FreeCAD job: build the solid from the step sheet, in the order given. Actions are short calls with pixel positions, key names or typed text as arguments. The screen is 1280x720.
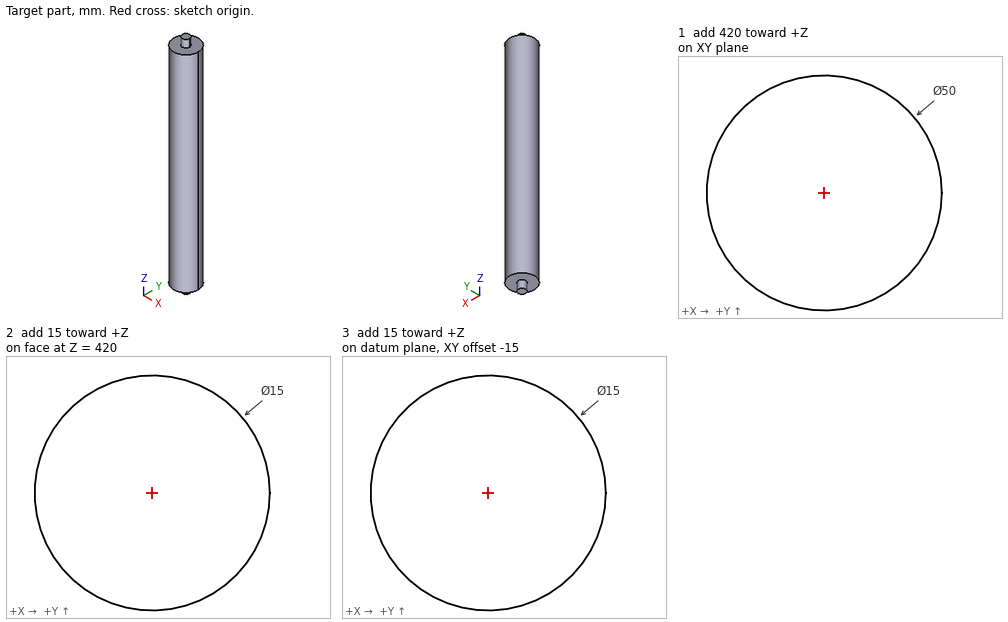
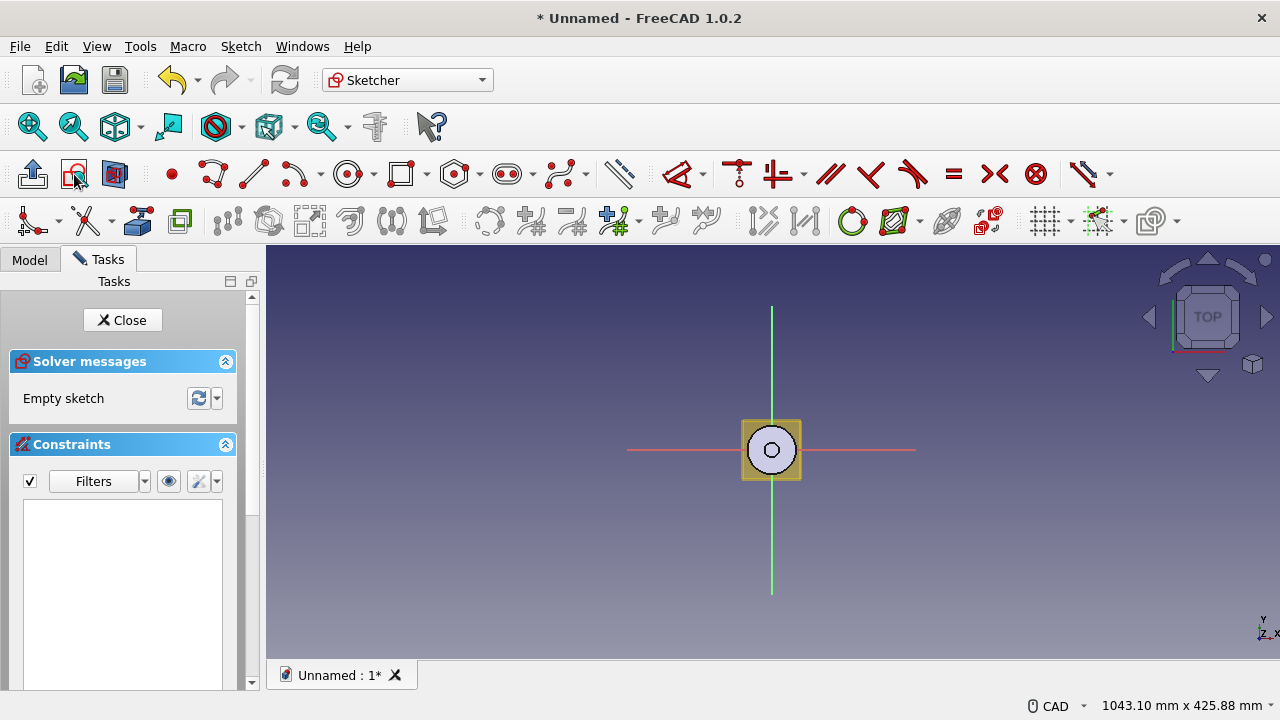
key(q)
key(s)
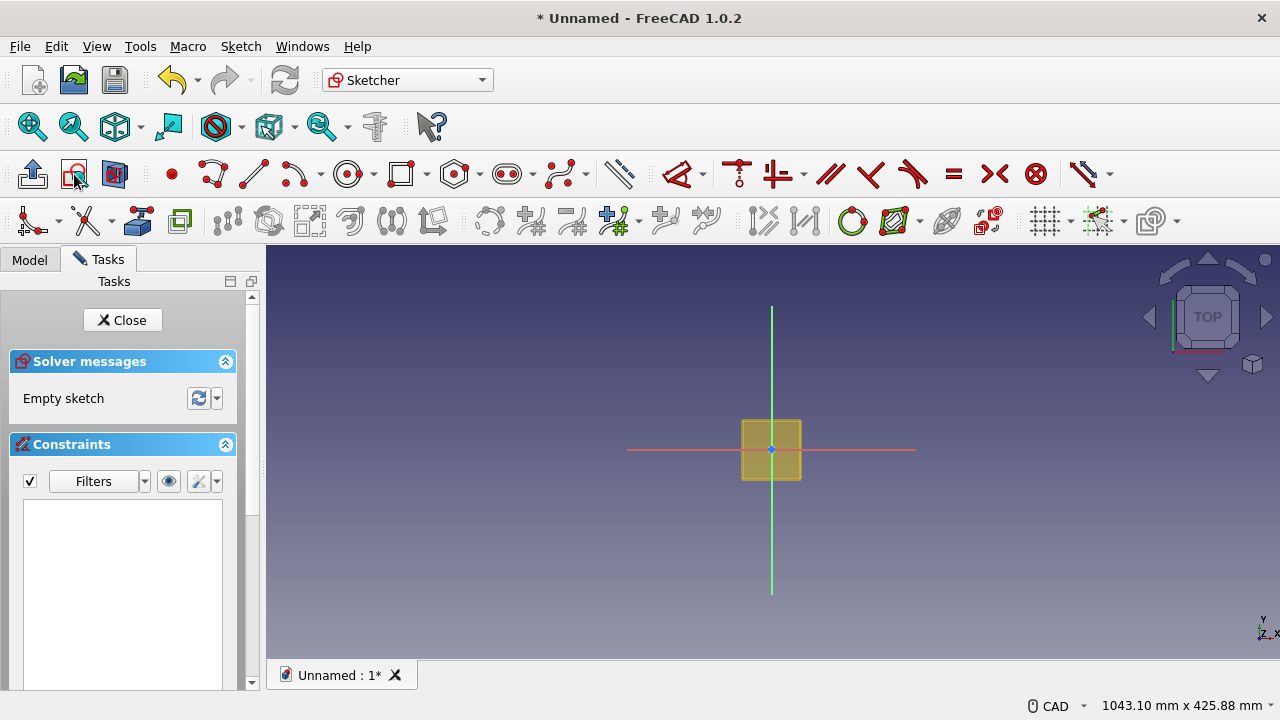
scroll(776, 450, up, 14)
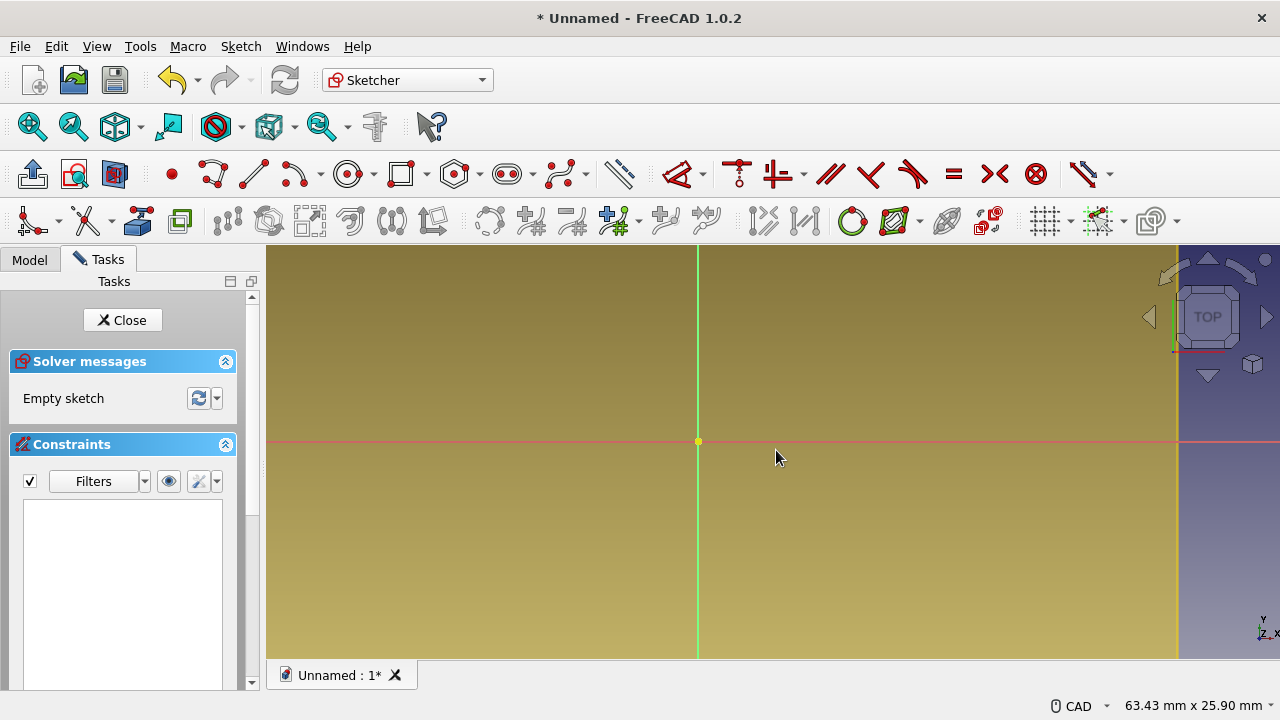
key(g)
key(c)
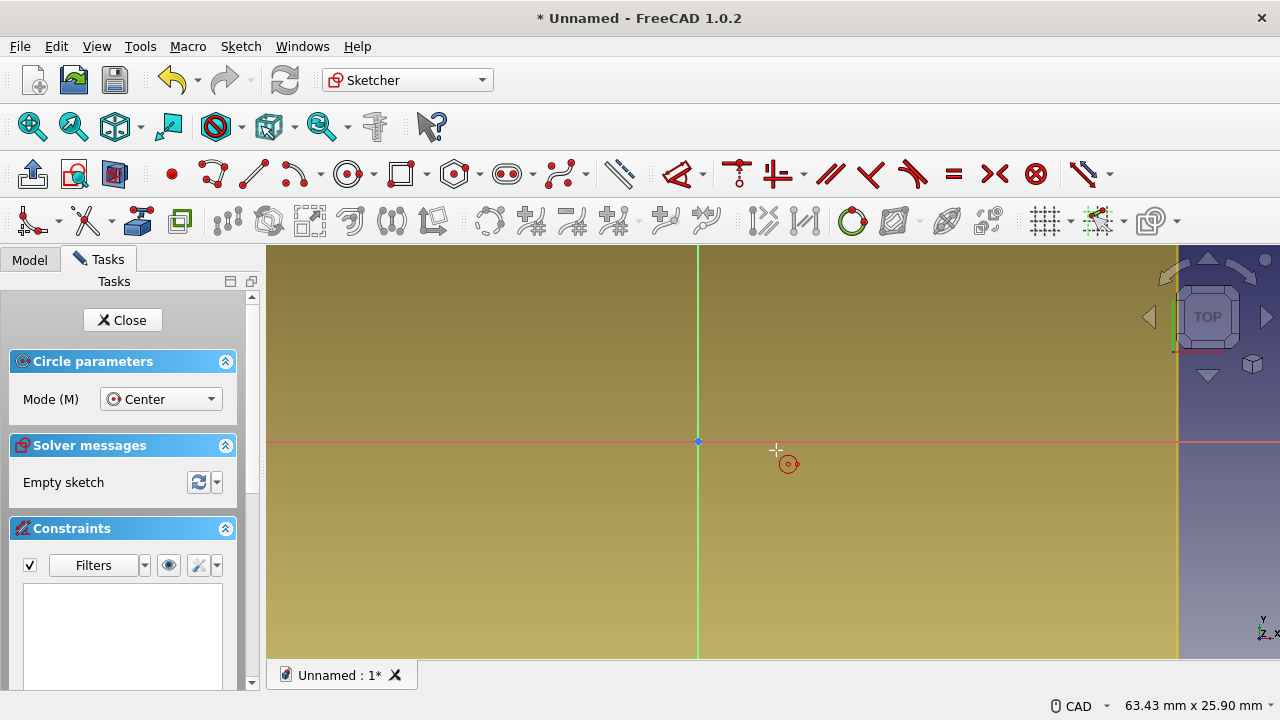
click(698, 442)
move(783, 357)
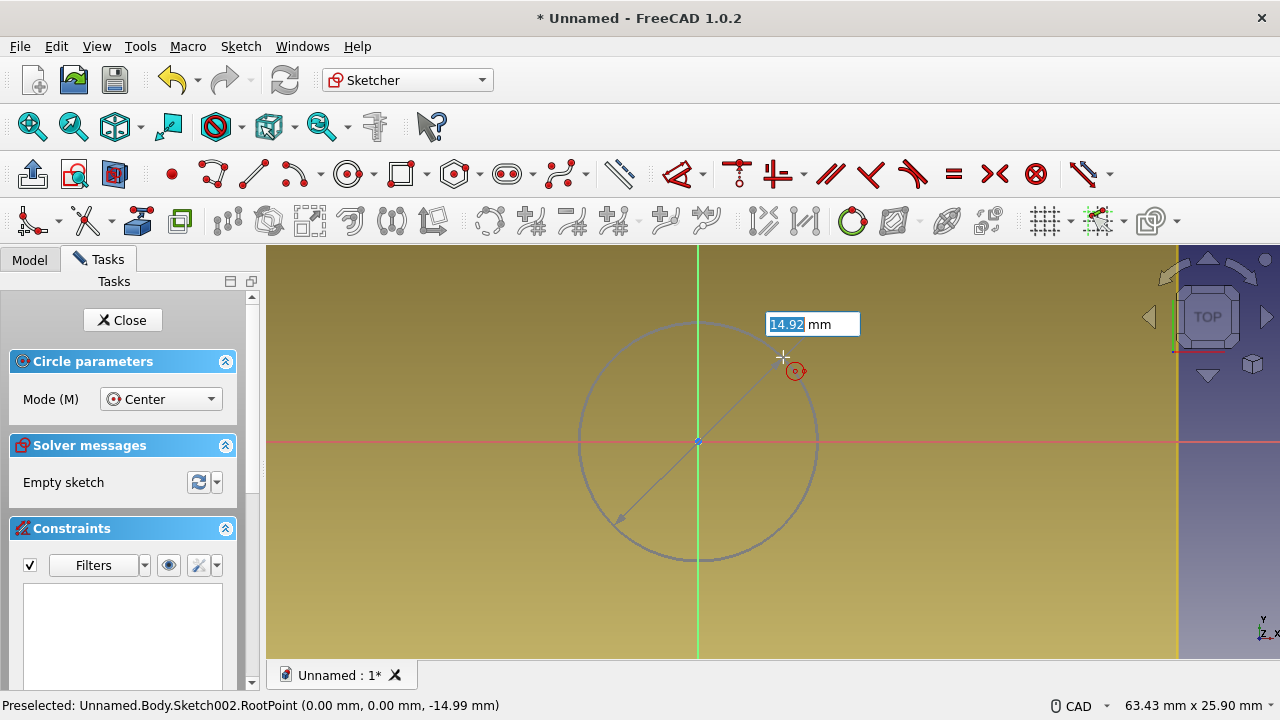
text(15)
key(Return)
key(Escape)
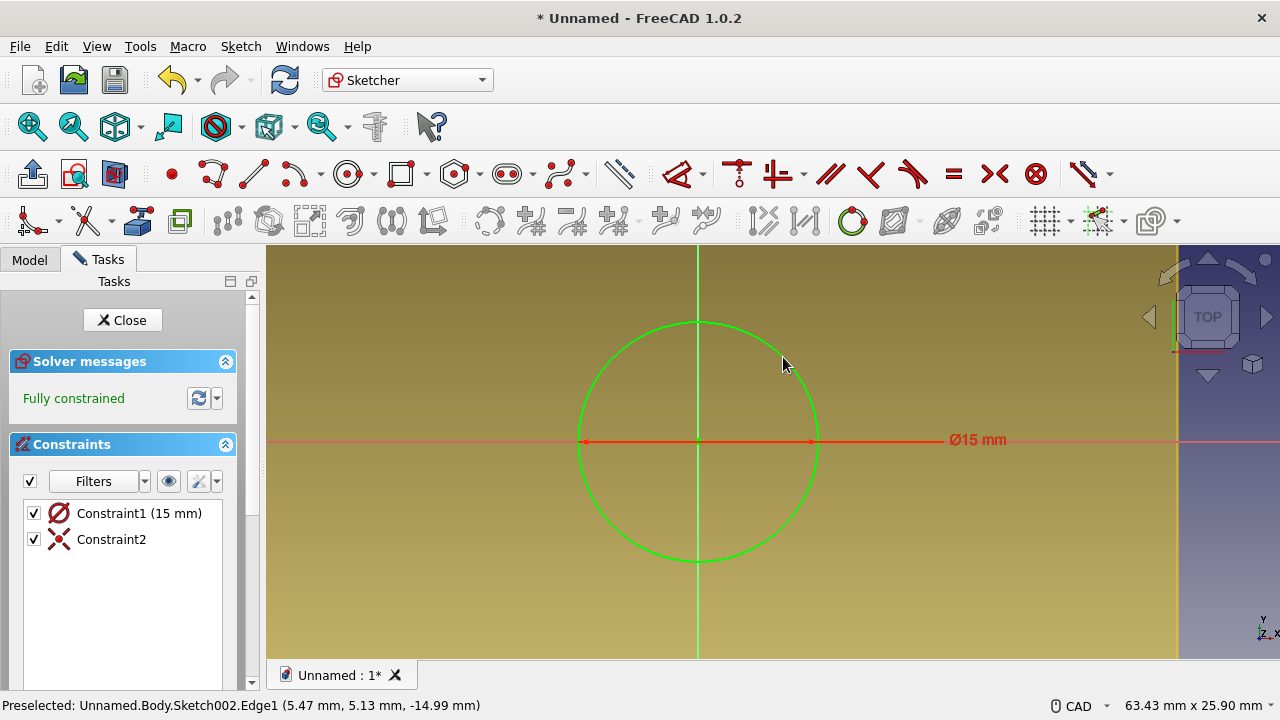
click(123, 320)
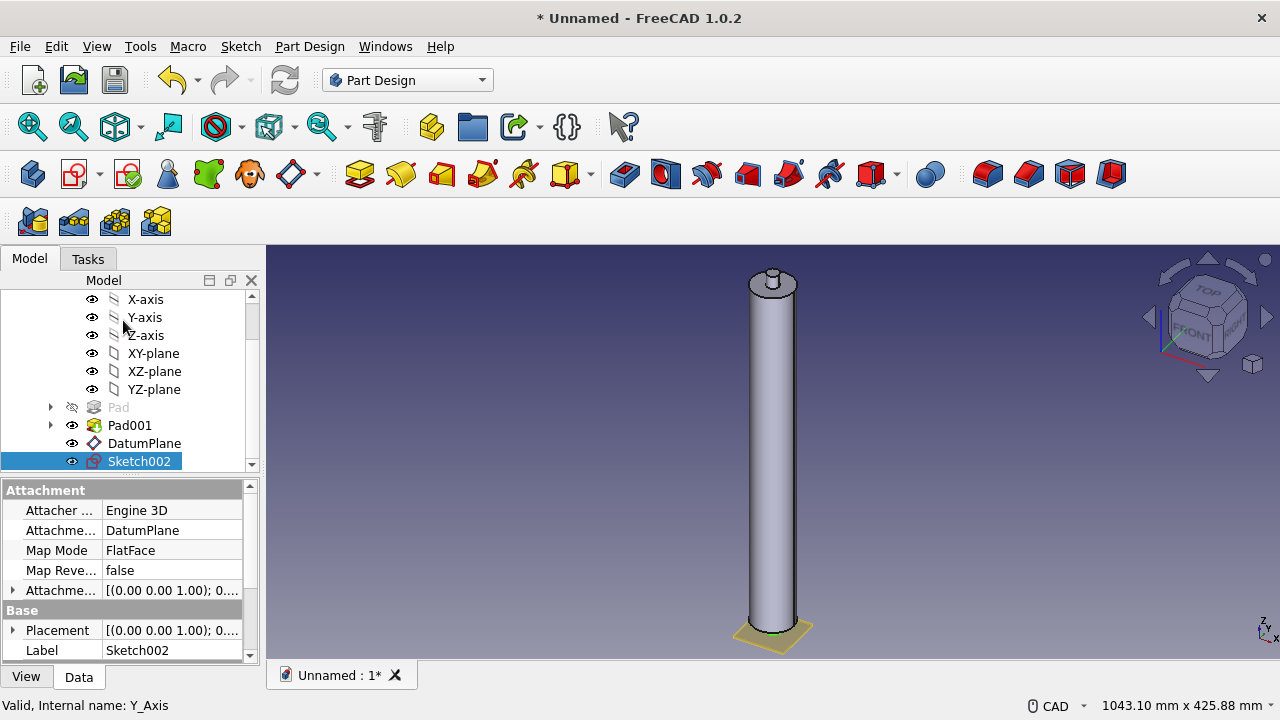
click(360, 174)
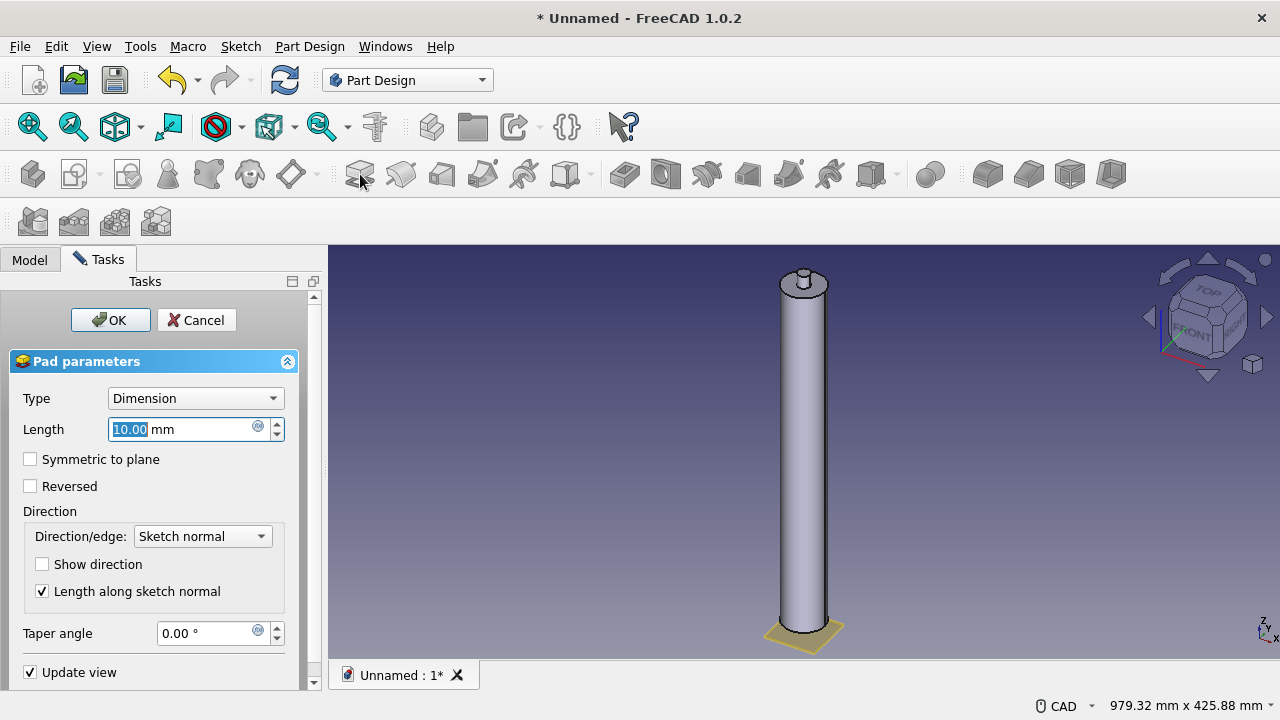
text(15)
key(Tab)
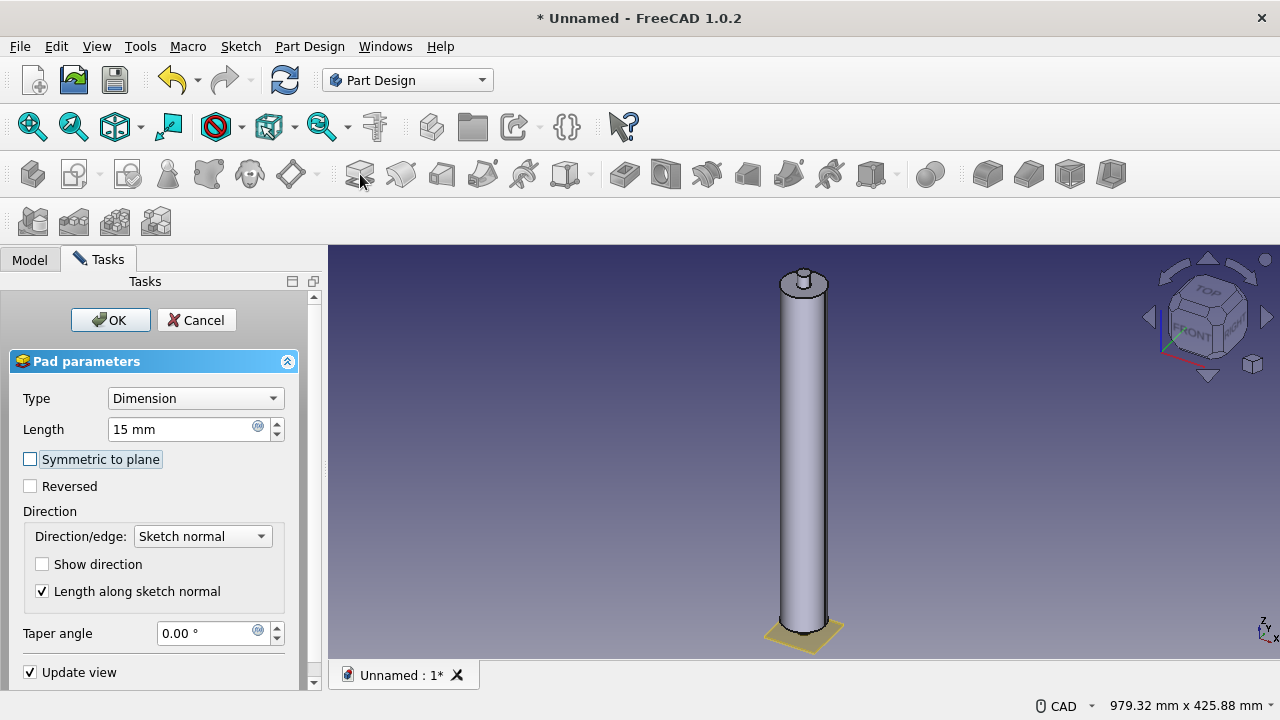
click(111, 320)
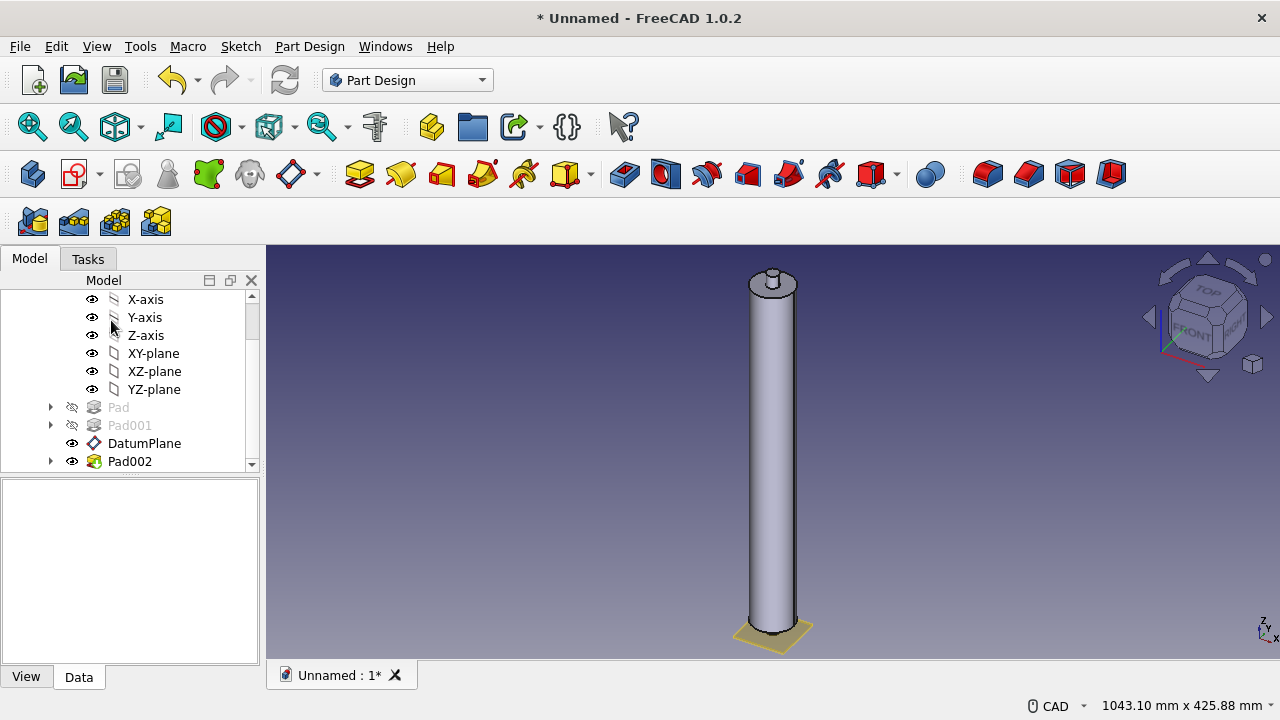
click(117, 443)
key(space)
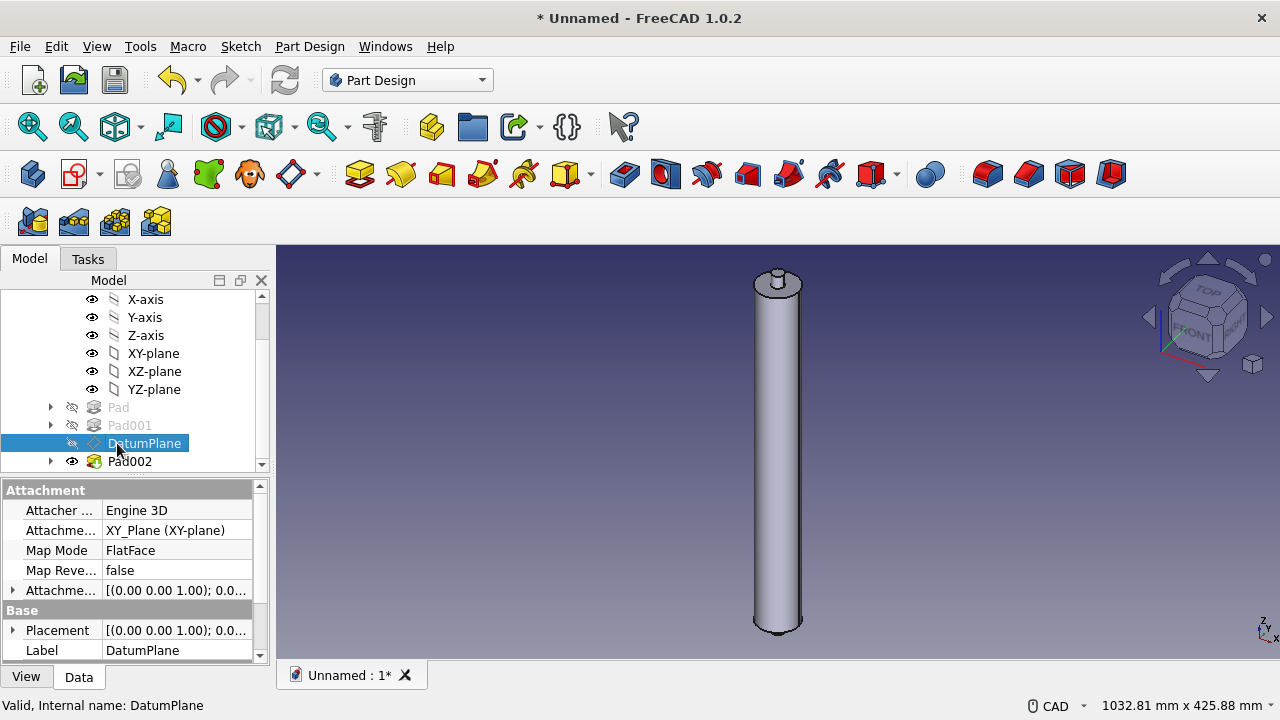
key(0)